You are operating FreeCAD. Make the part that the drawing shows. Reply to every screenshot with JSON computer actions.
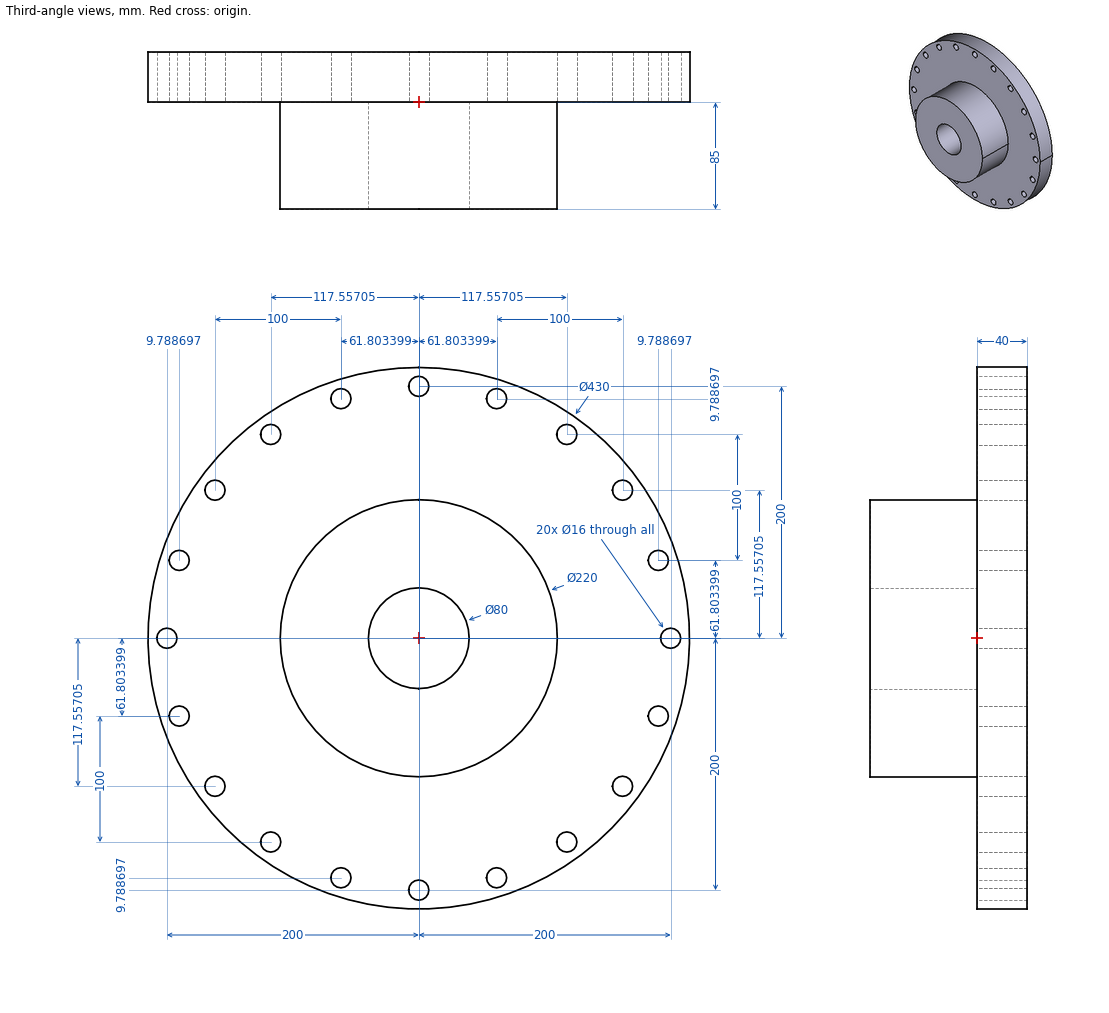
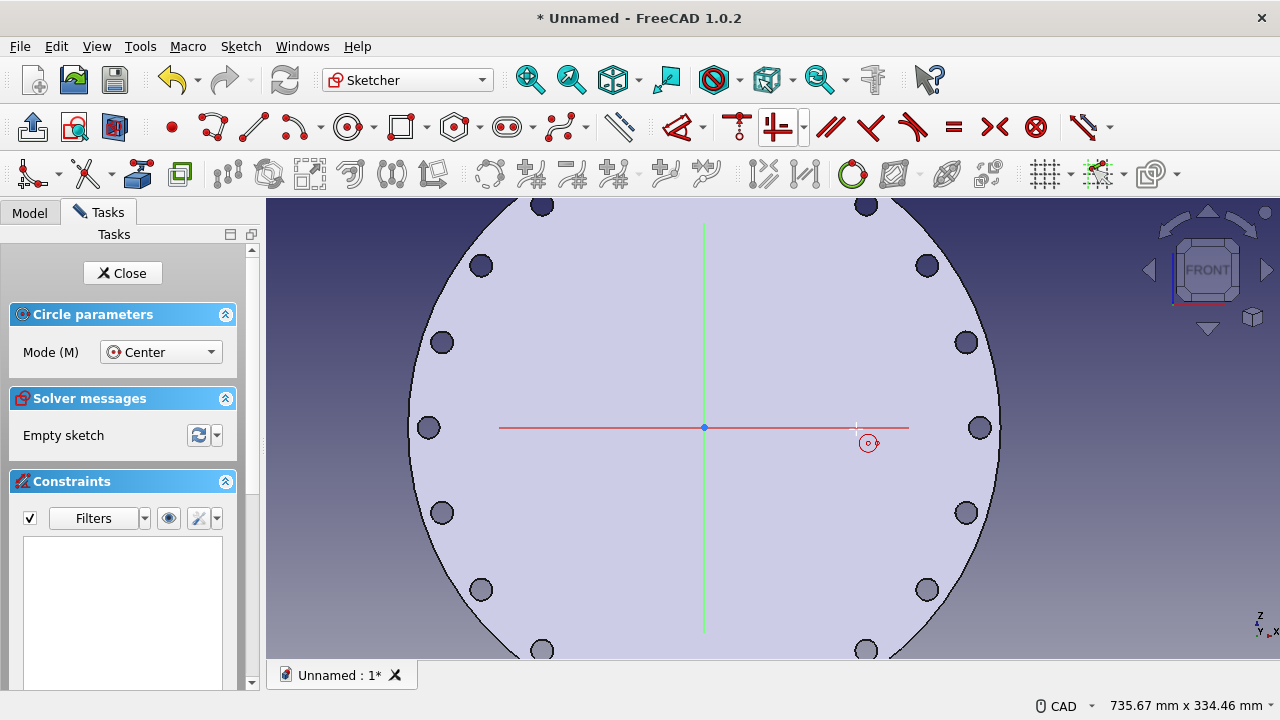
{"action": "left_click", "coordinate": [704, 428]}
{"action": "left_click", "coordinate": [811, 320]}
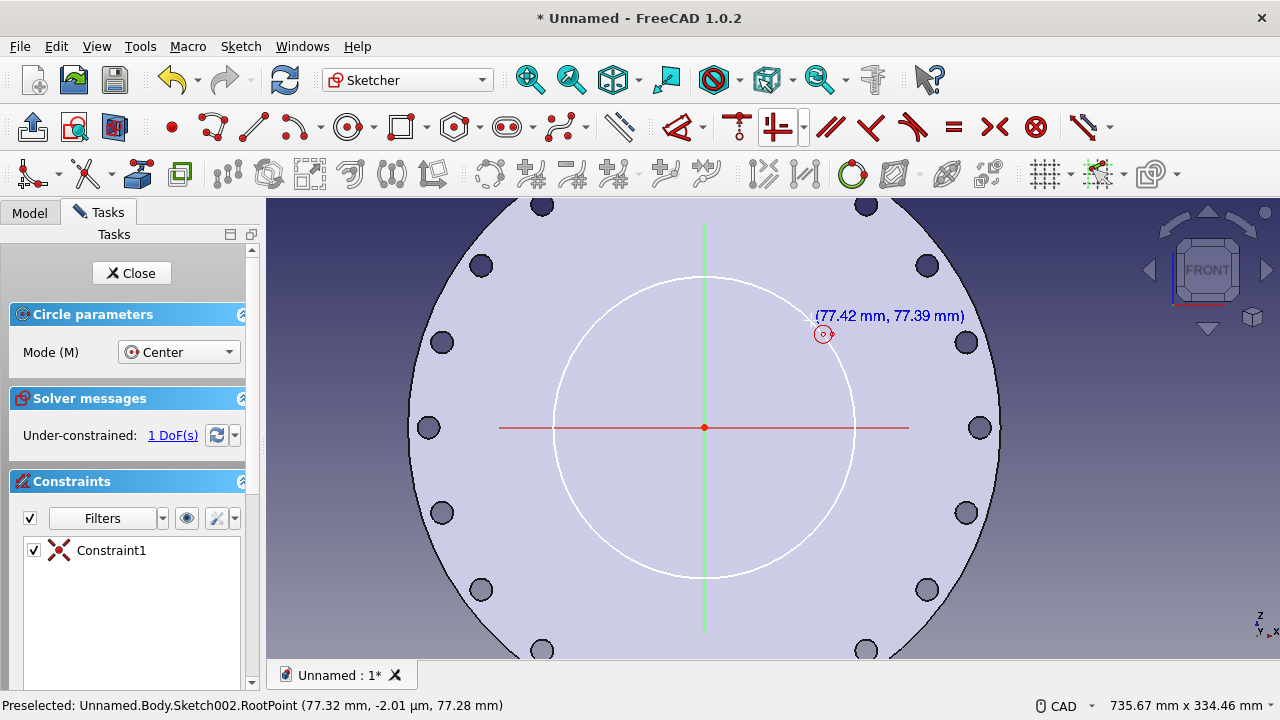
{"action": "left_click", "coordinate": [704, 428]}
{"action": "left_click", "coordinate": [743, 389]}
{"action": "key", "text": "Escape"}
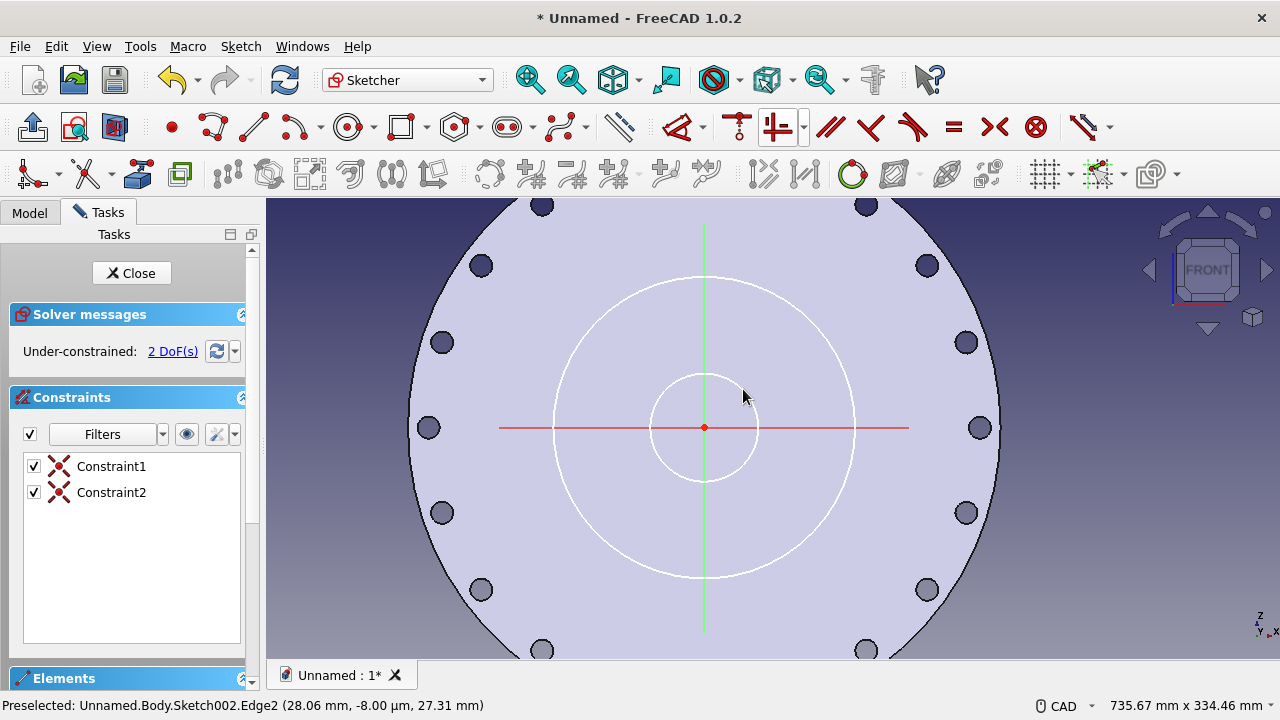
{"action": "key", "text": "d"}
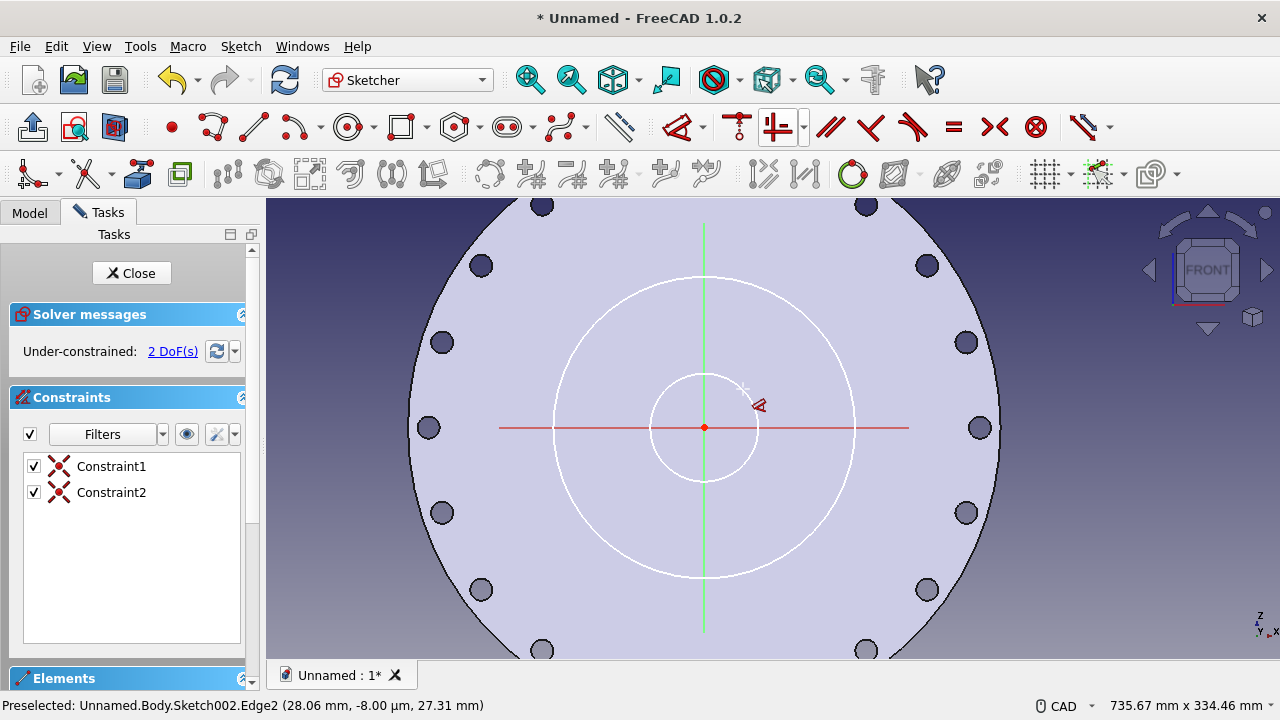
{"action": "left_click", "coordinate": [811, 321]}
{"action": "left_click", "coordinate": [834, 298]}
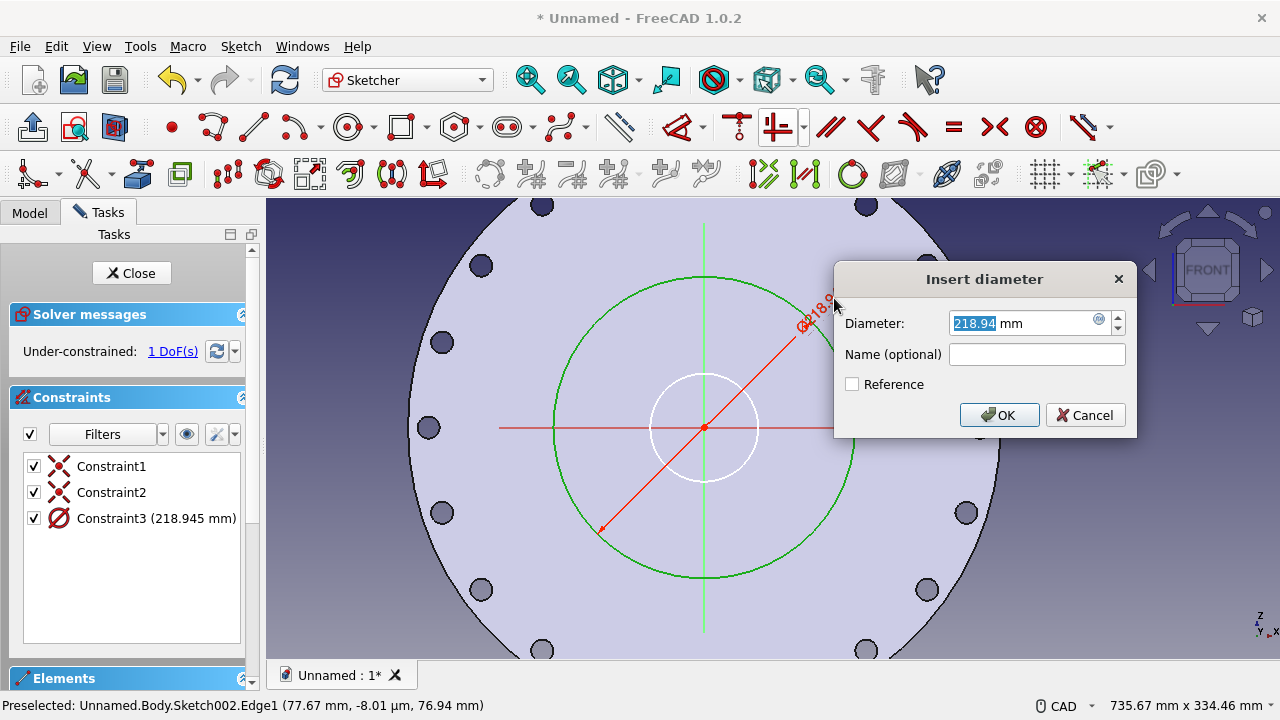
{"action": "type", "text": "220"}
{"action": "key", "text": "Return"}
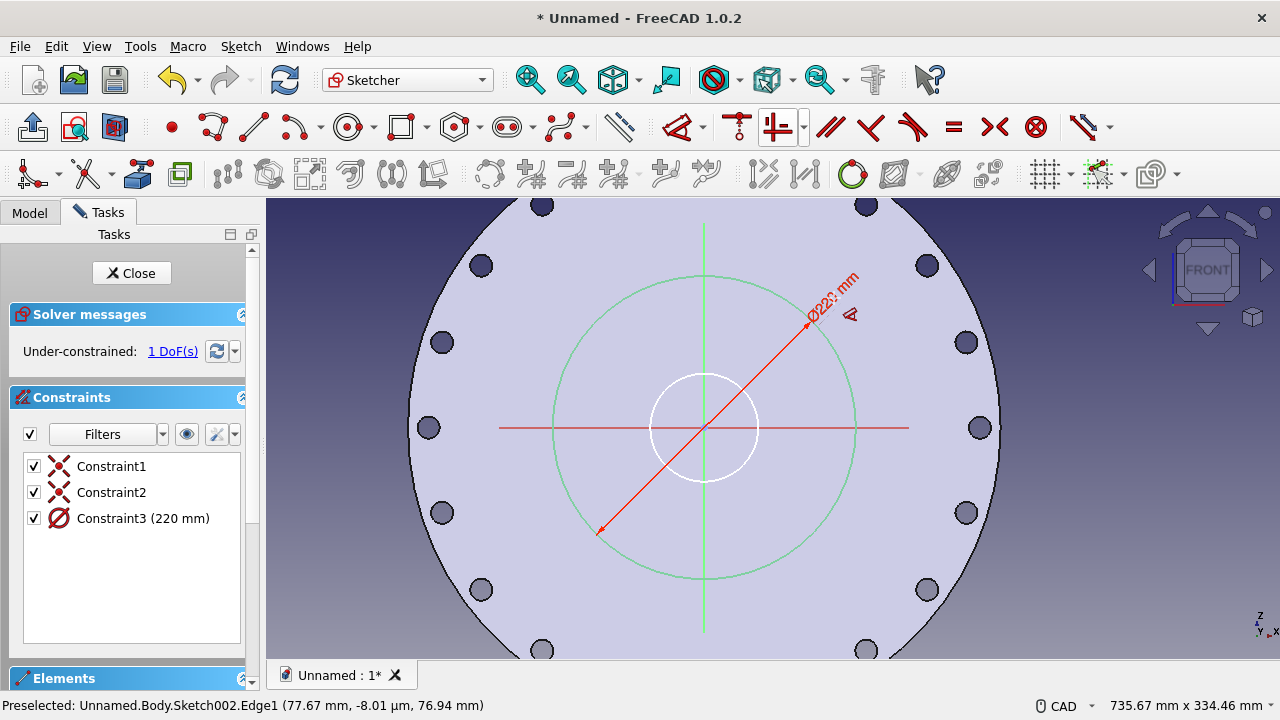
{"action": "left_click", "coordinate": [742, 389]}
{"action": "left_click", "coordinate": [764, 366]}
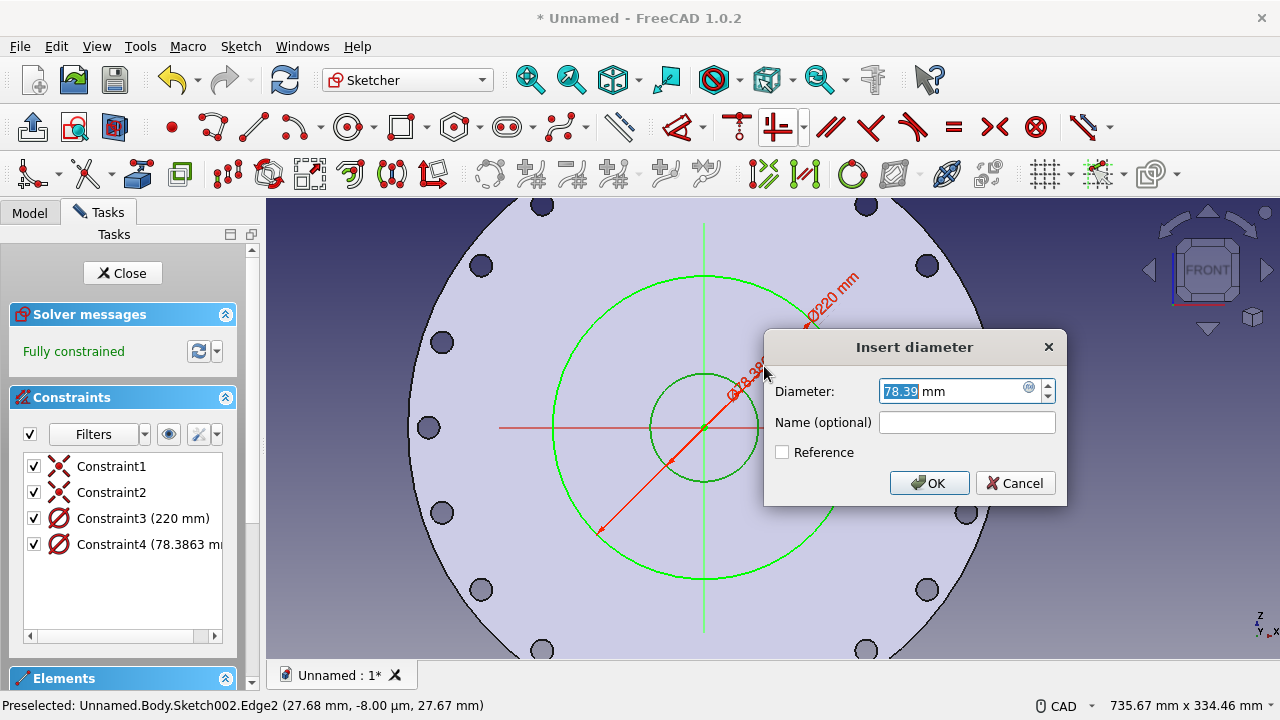
{"action": "type", "text": "80"}
{"action": "key", "text": "Return"}
{"action": "key", "text": "Escape"}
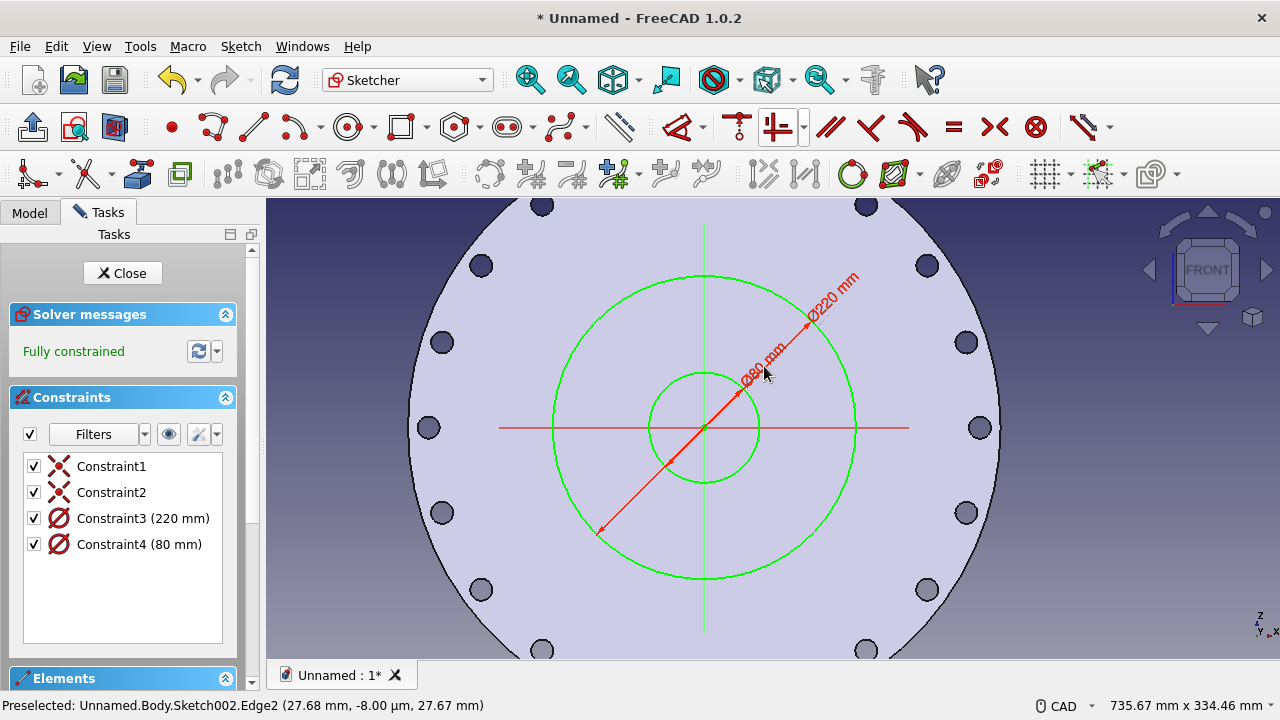
{"action": "left_click", "coordinate": [123, 273]}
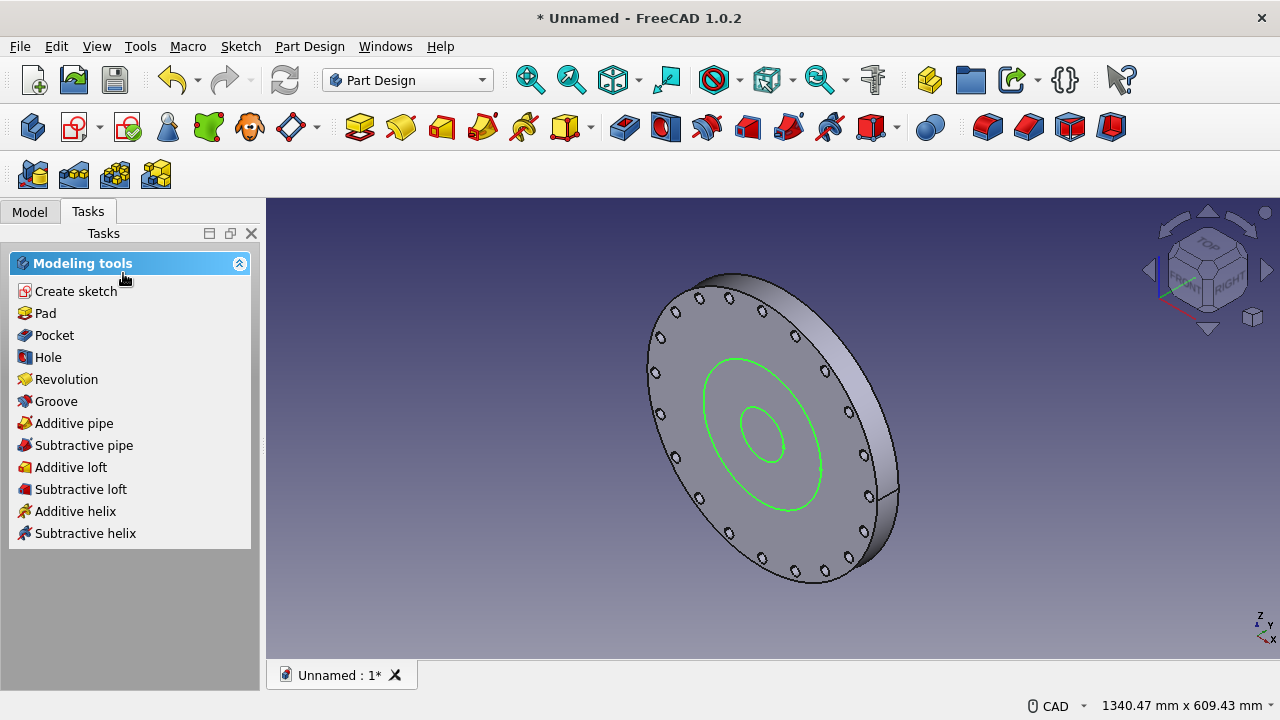
{"action": "left_click", "coordinate": [360, 128]}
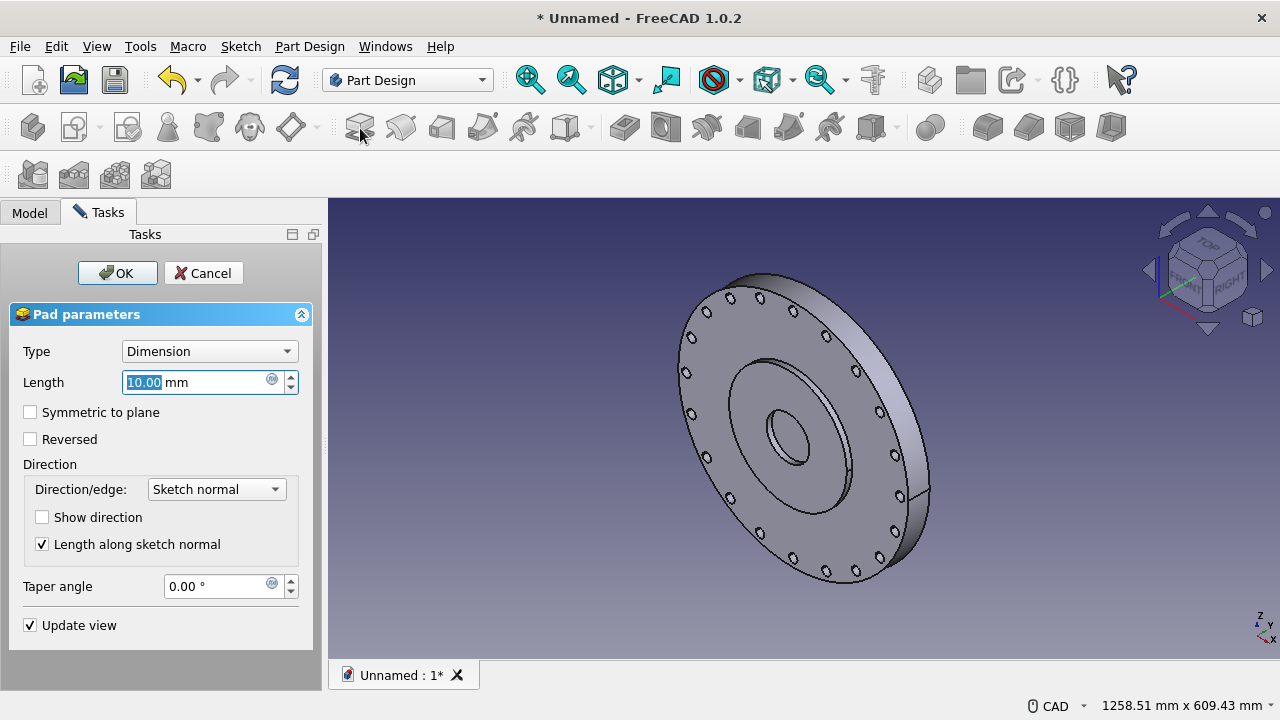
{"action": "type", "text": "85"}
{"action": "key", "text": "Tab"}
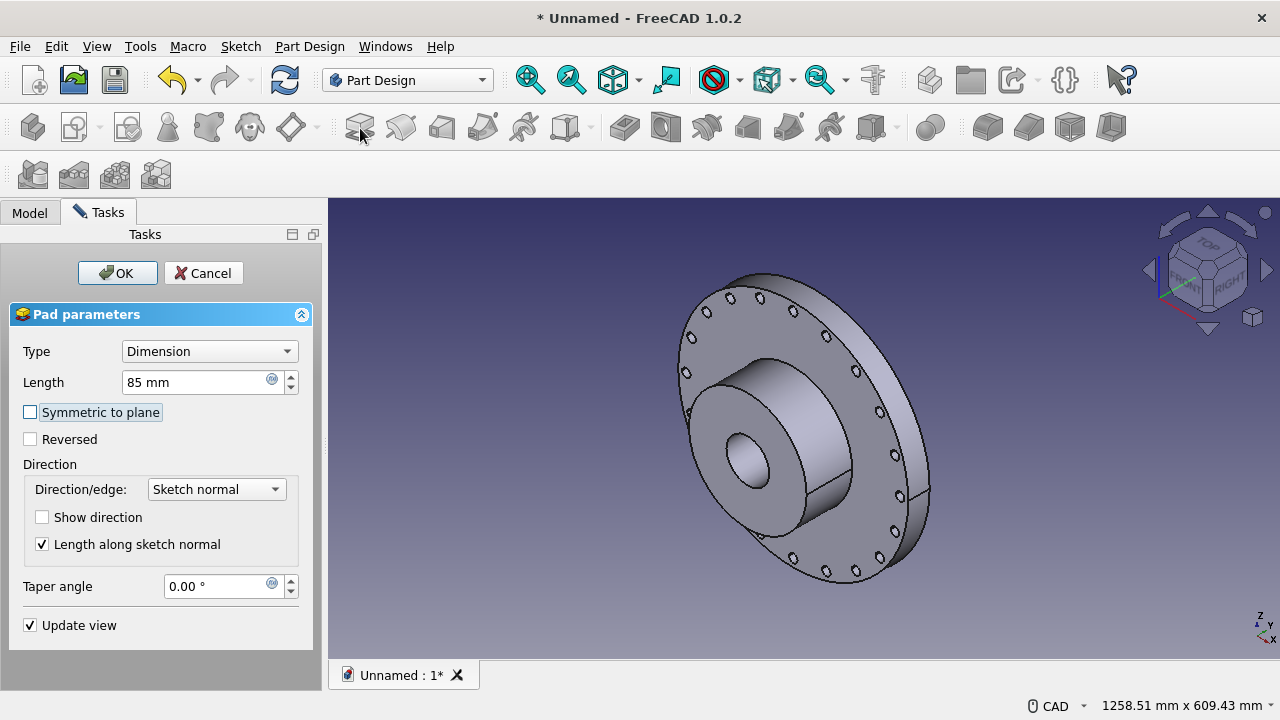
{"action": "left_click", "coordinate": [118, 273]}